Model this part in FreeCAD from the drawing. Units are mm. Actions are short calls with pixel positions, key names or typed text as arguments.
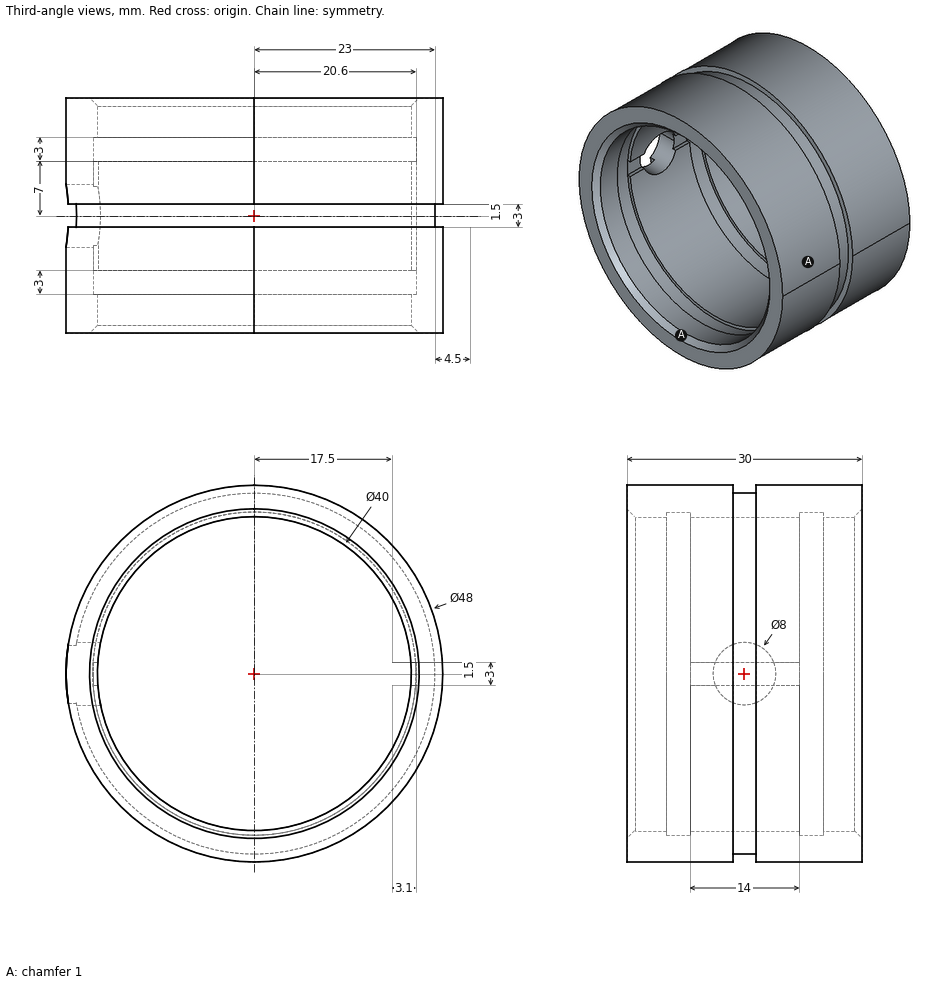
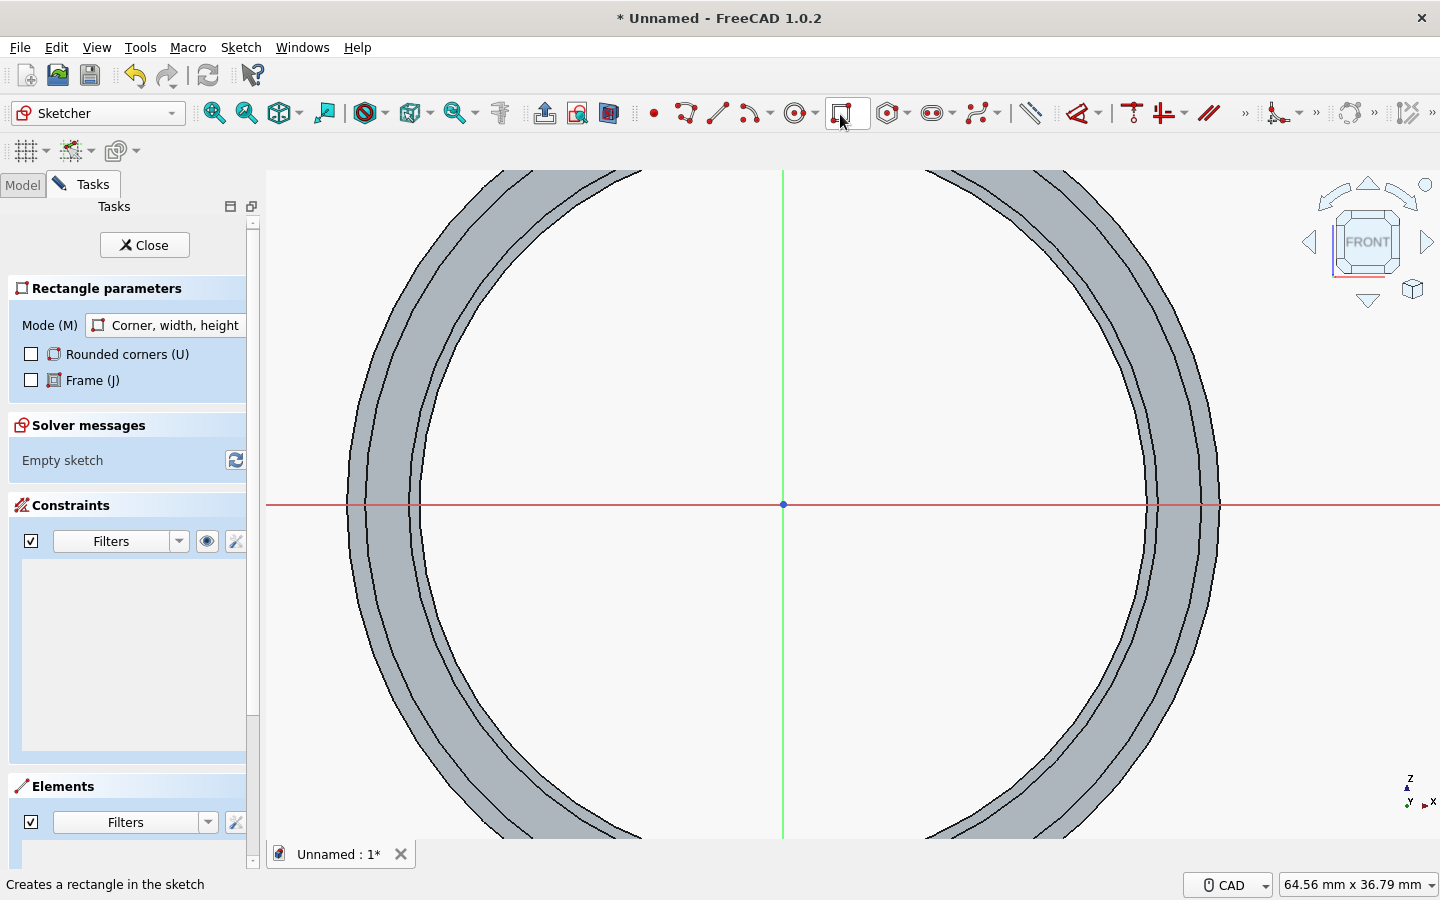
click(1102, 477)
click(1158, 532)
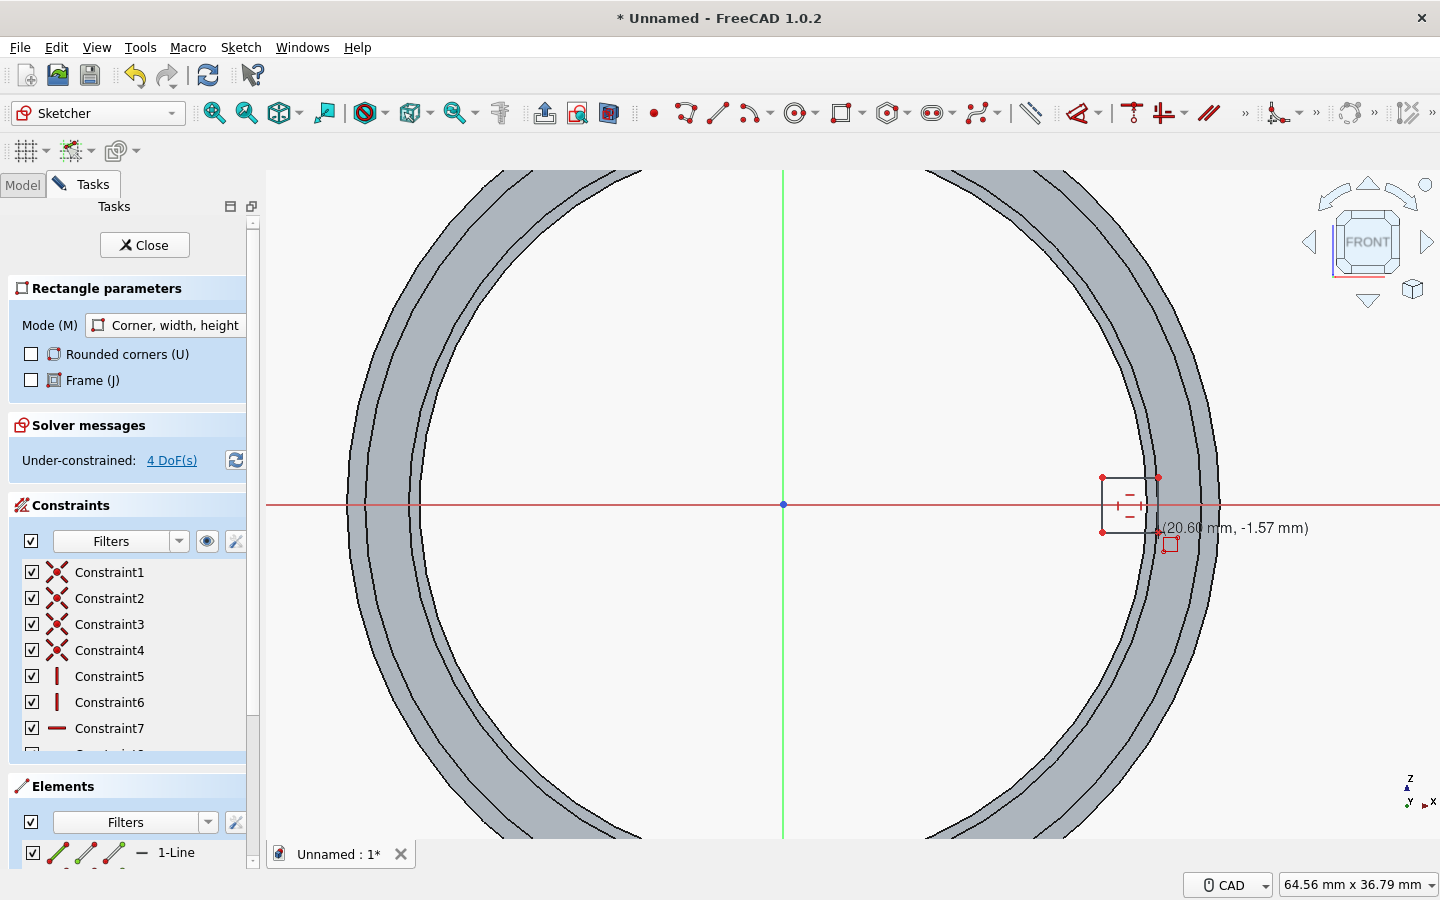
click(409, 477)
click(465, 532)
key(Escape)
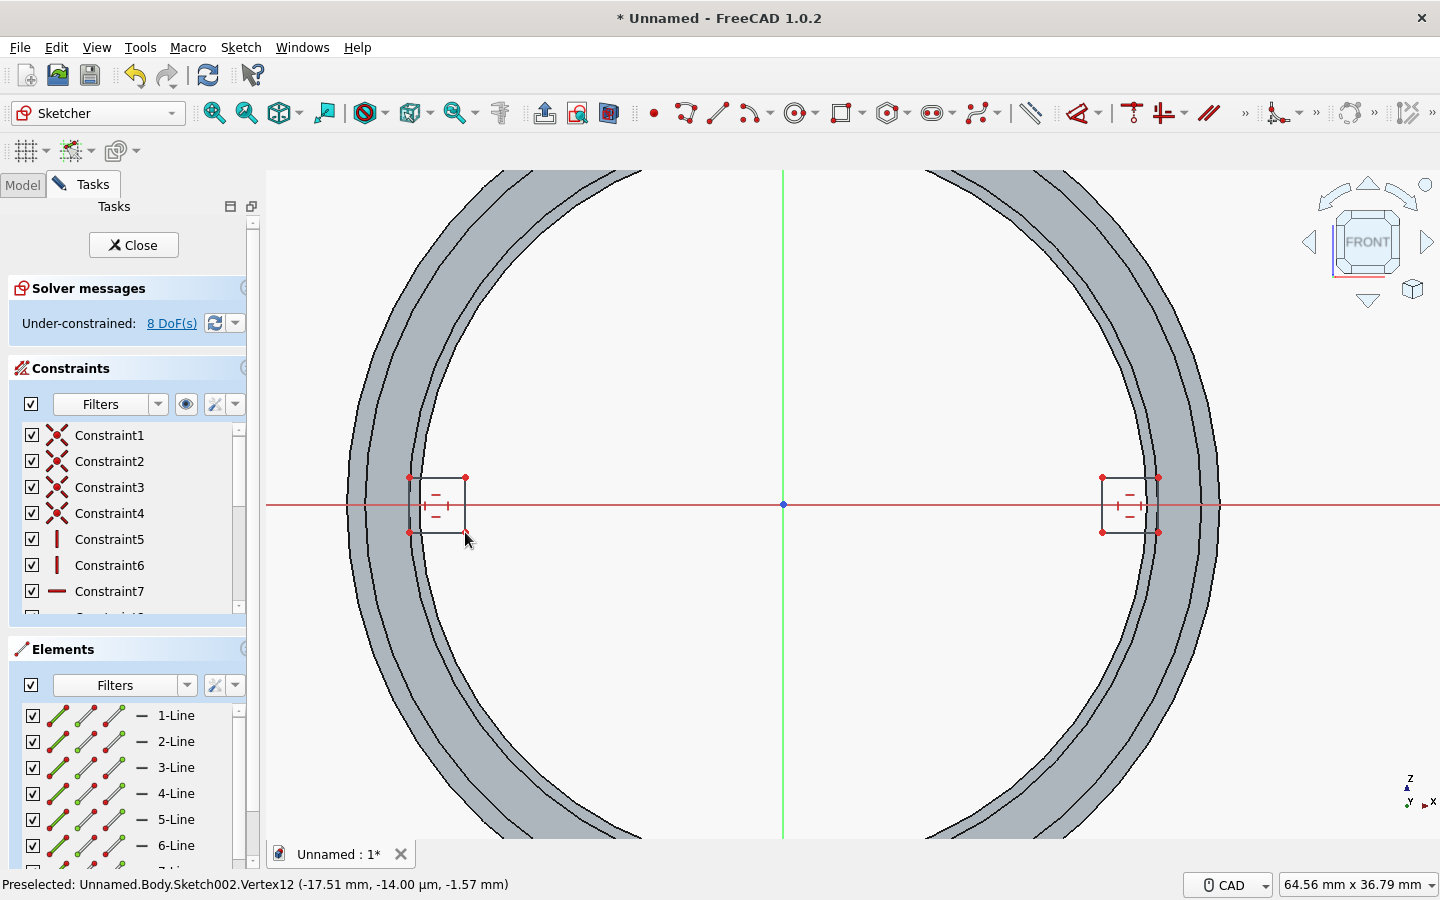
click(1158, 478)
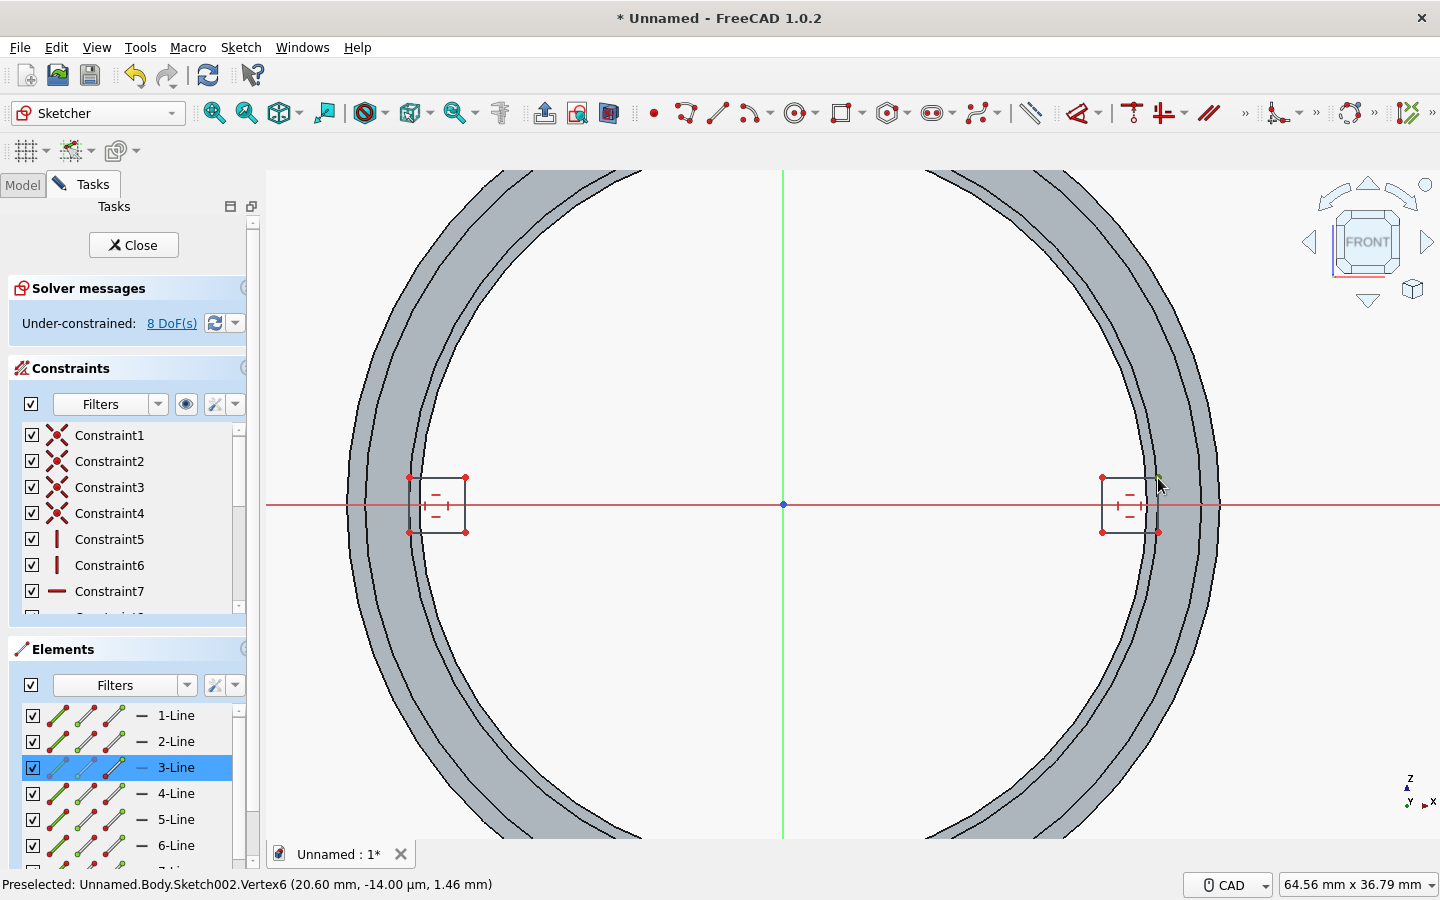
click(409, 478)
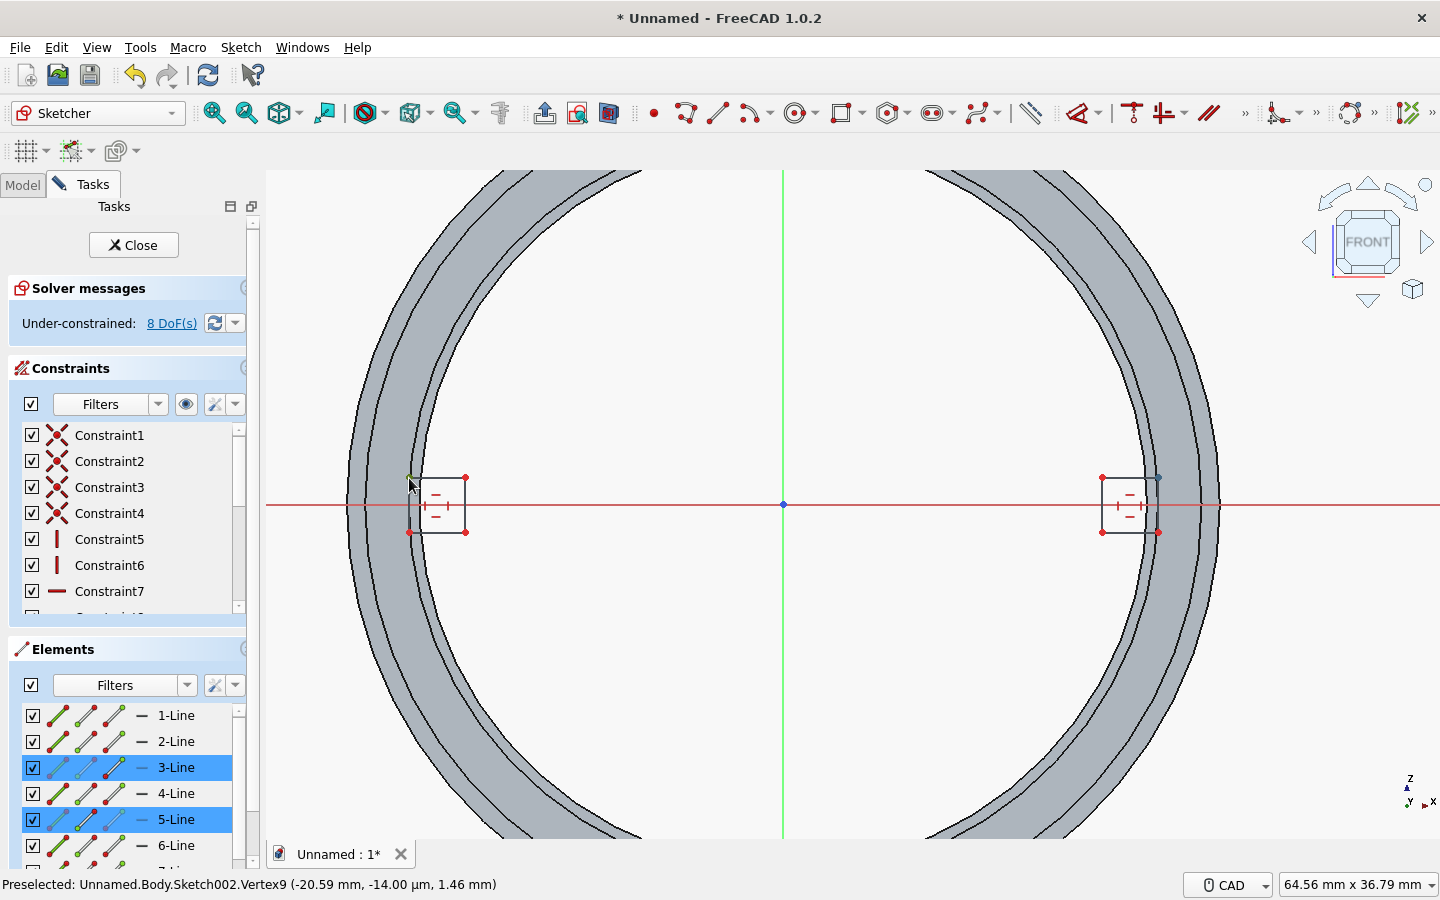
click(783, 767)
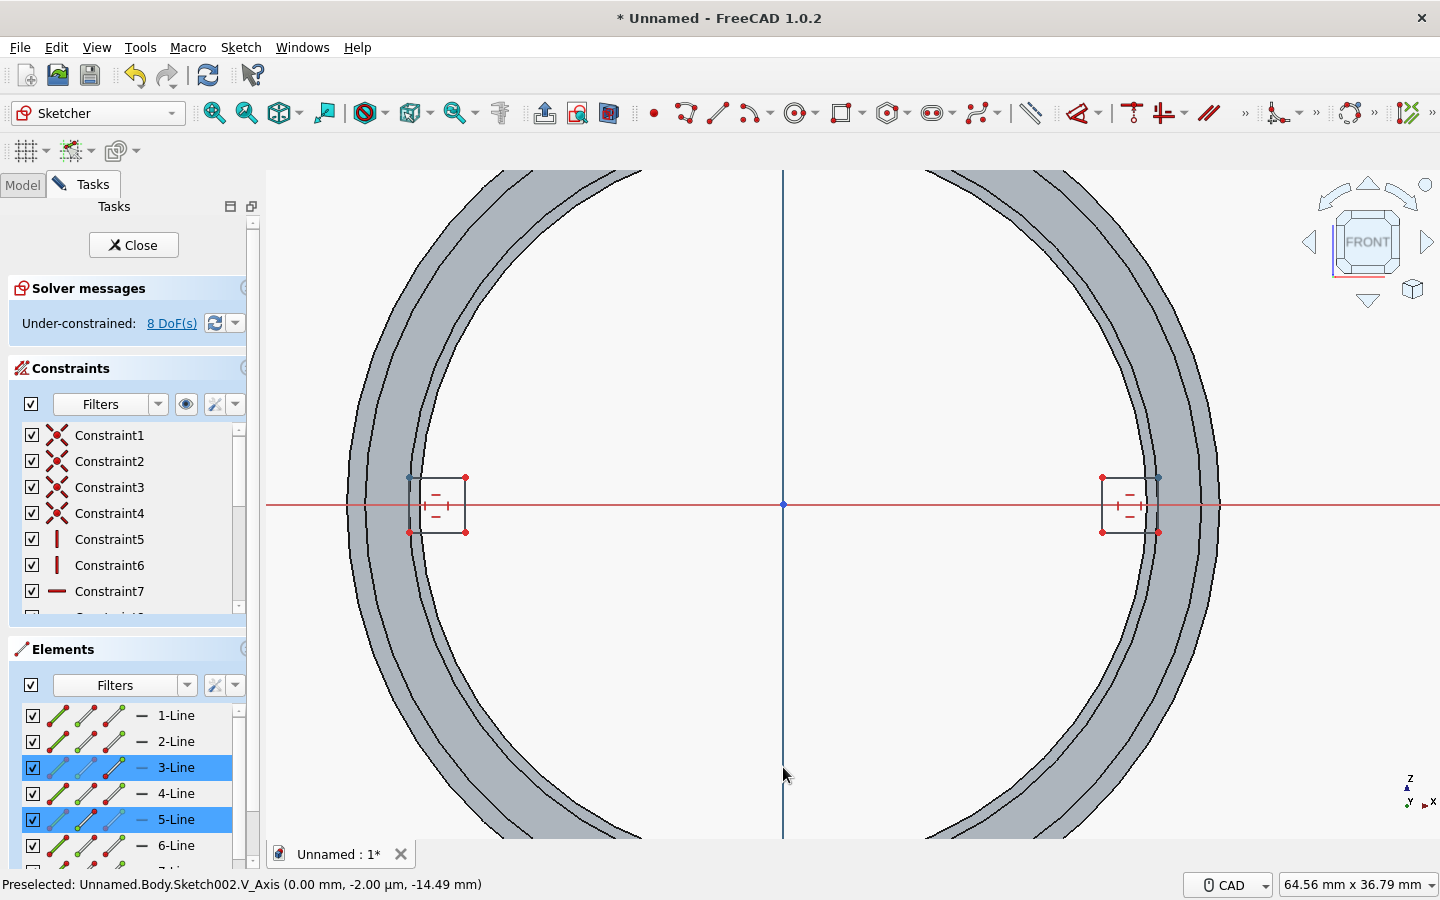
key(s)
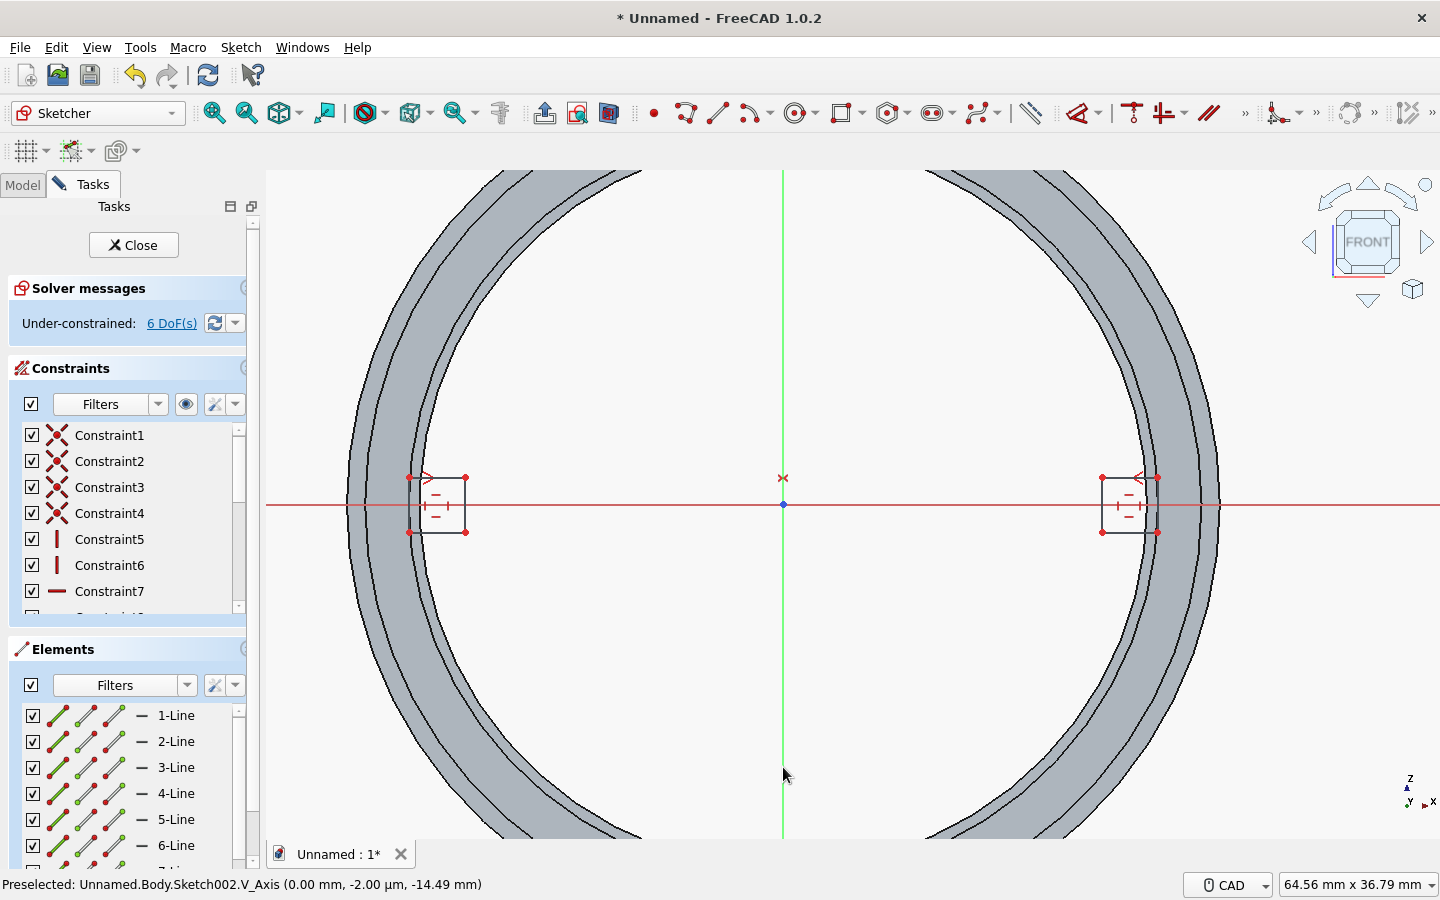
click(1102, 533)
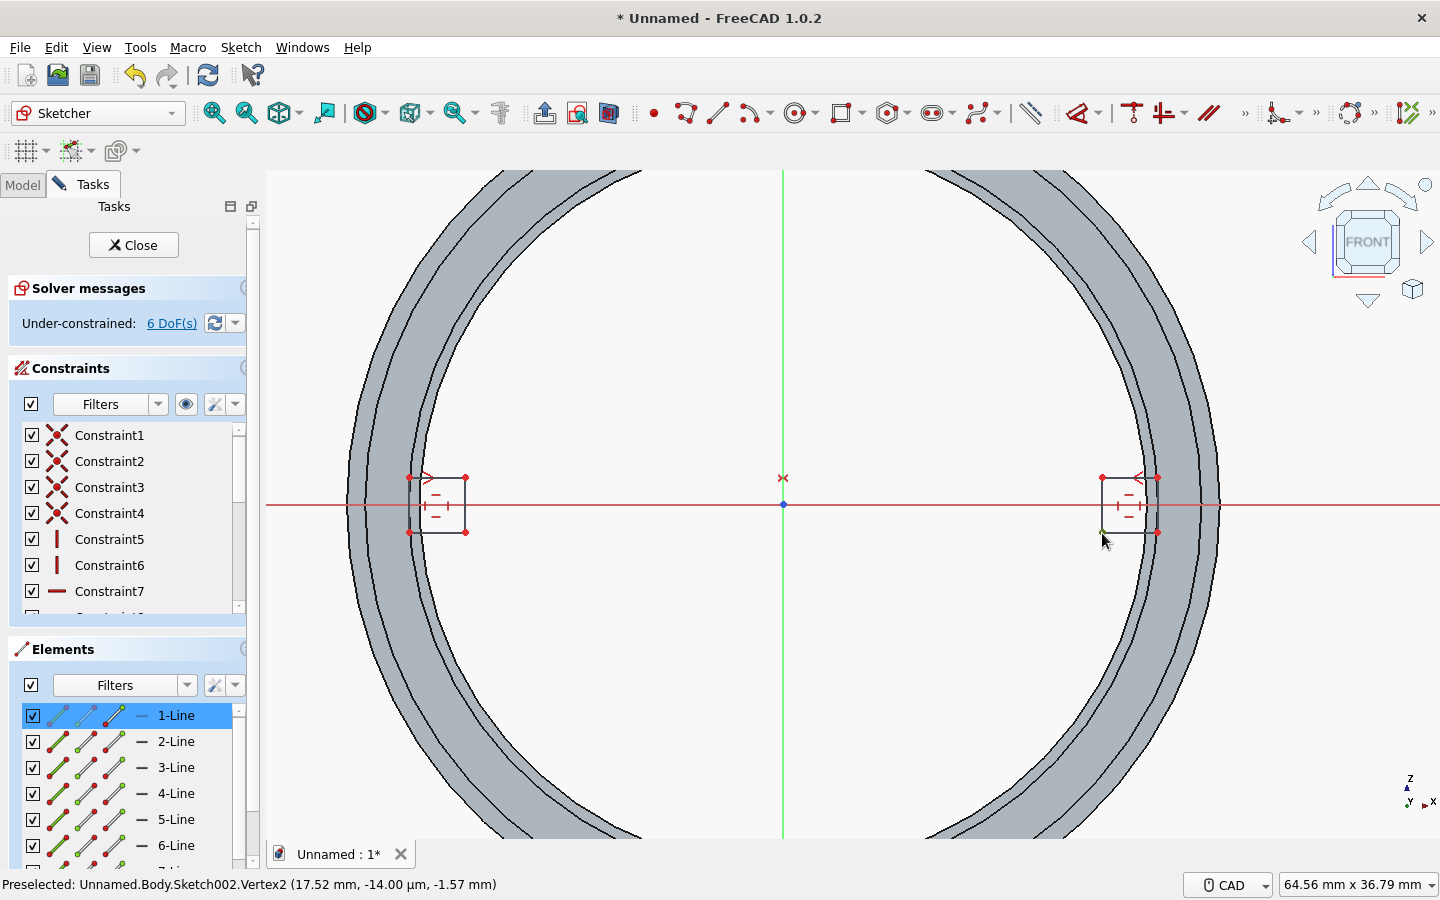
click(465, 533)